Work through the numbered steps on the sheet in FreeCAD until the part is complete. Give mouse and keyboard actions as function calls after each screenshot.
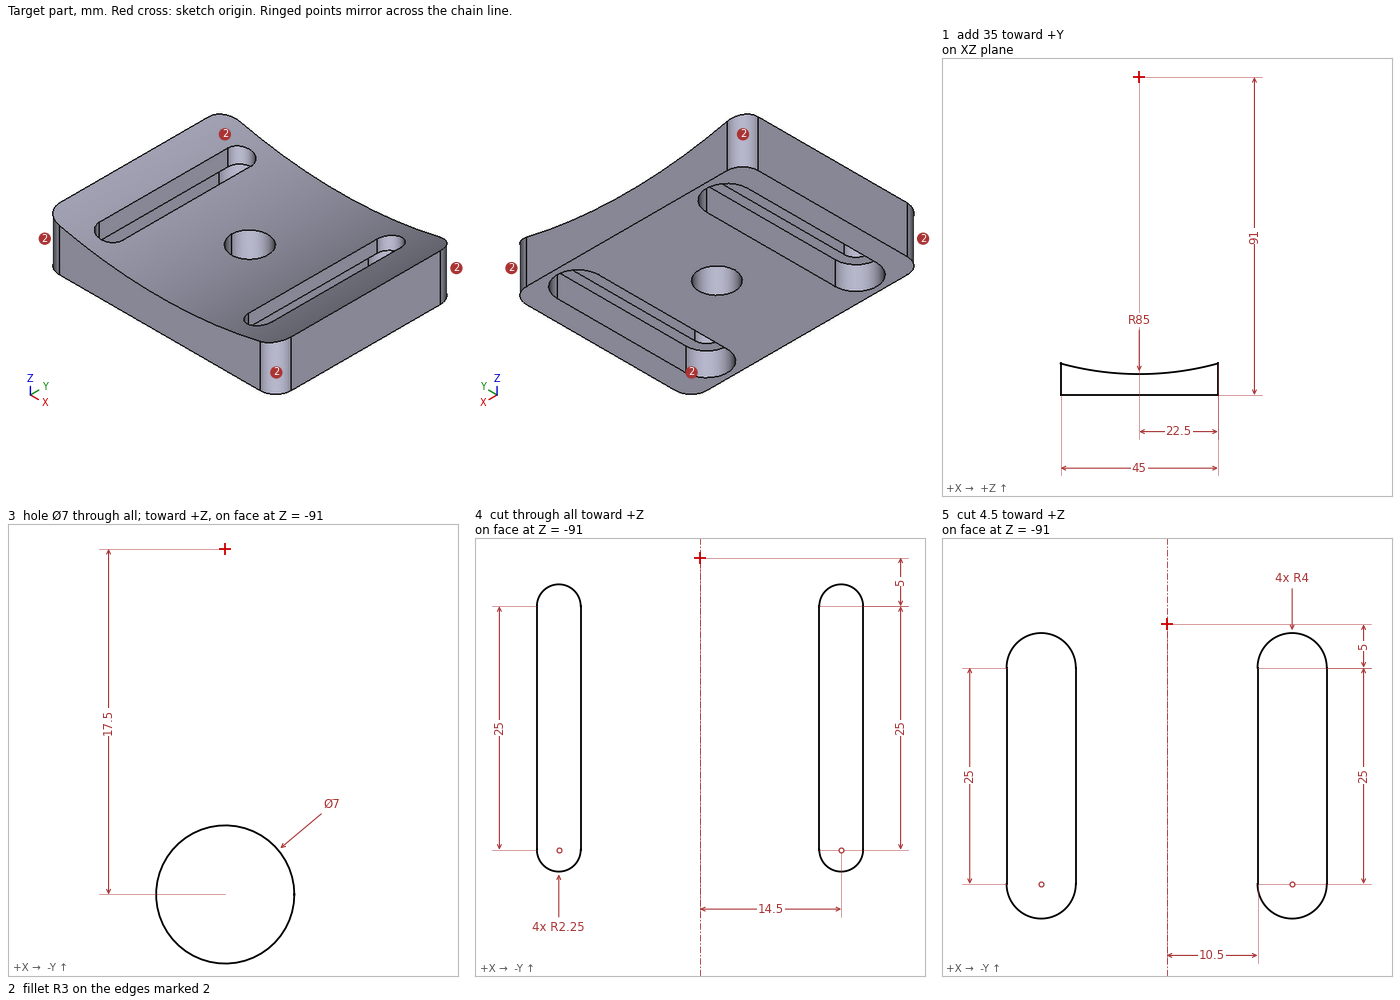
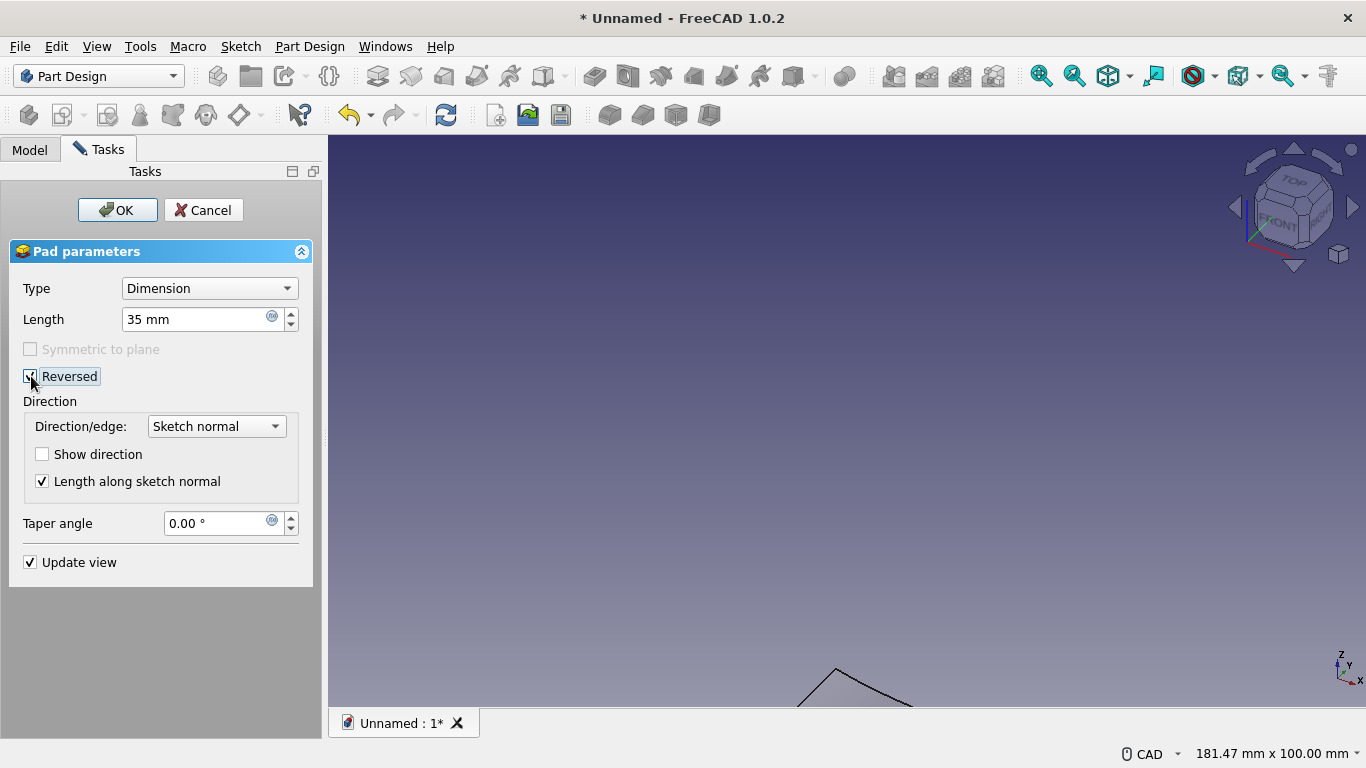
click(118, 210)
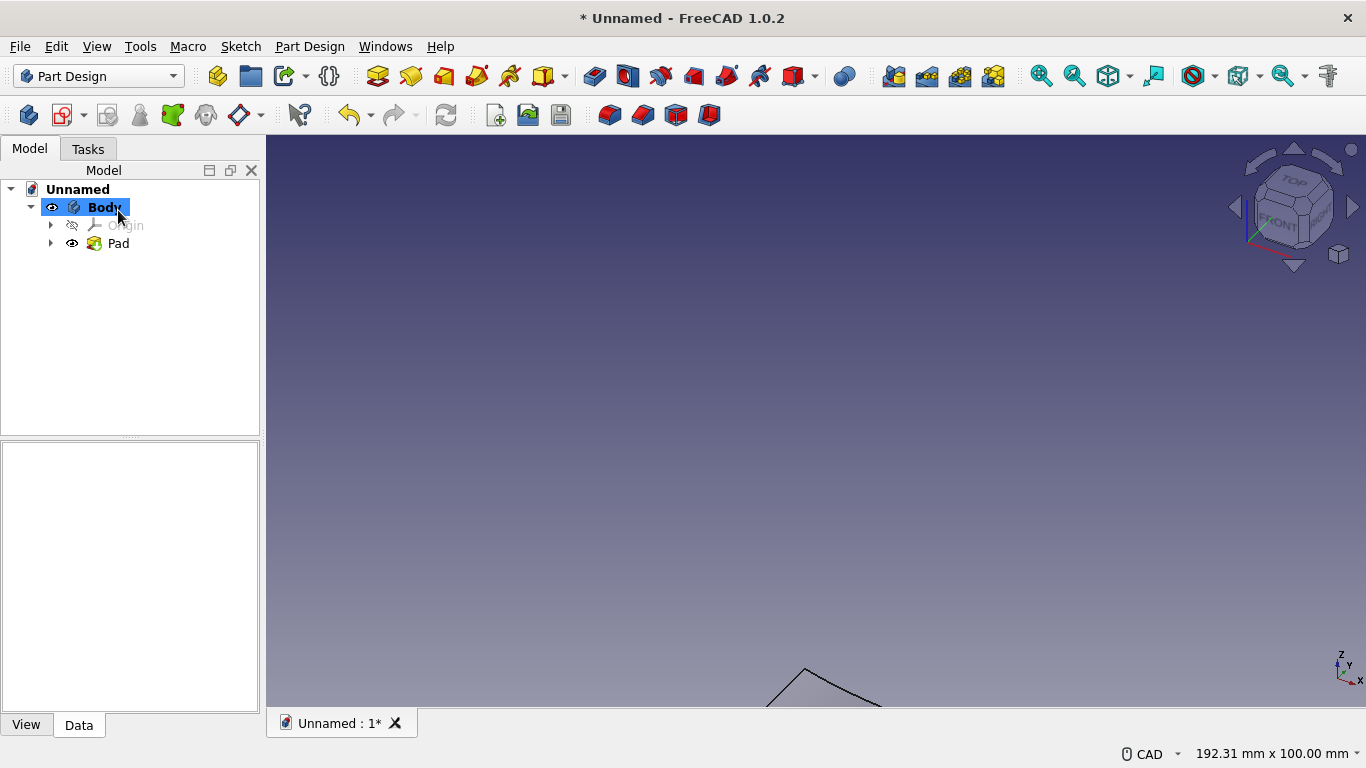
key(v)
key(f)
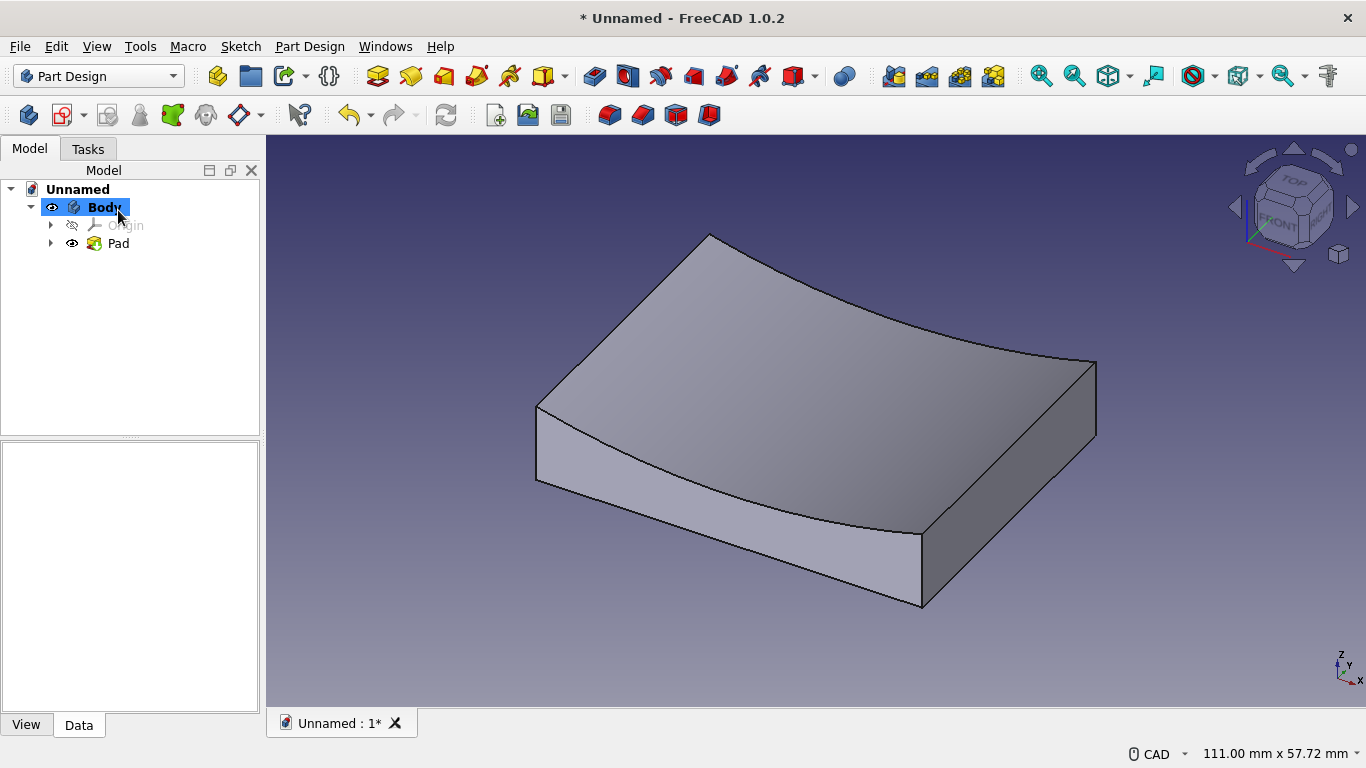
click(922, 570)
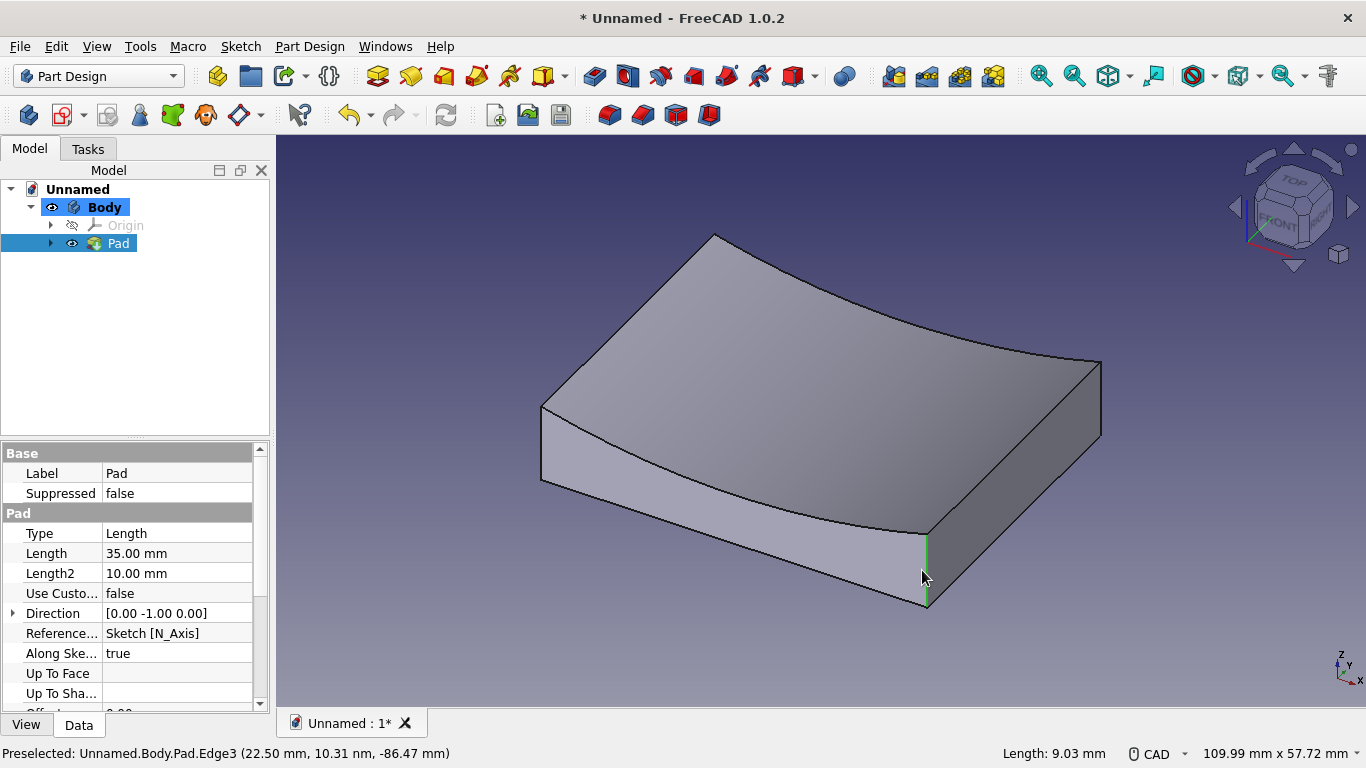
key(0)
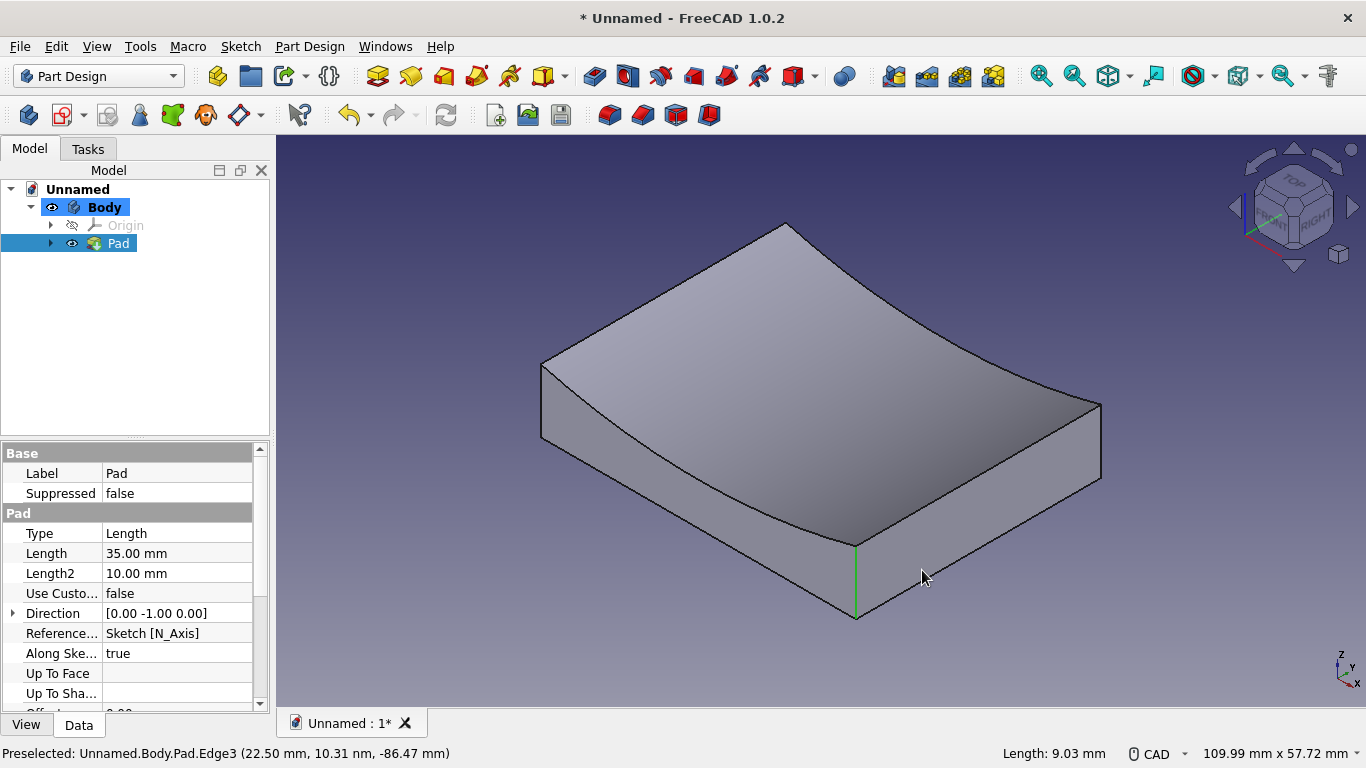
key(2)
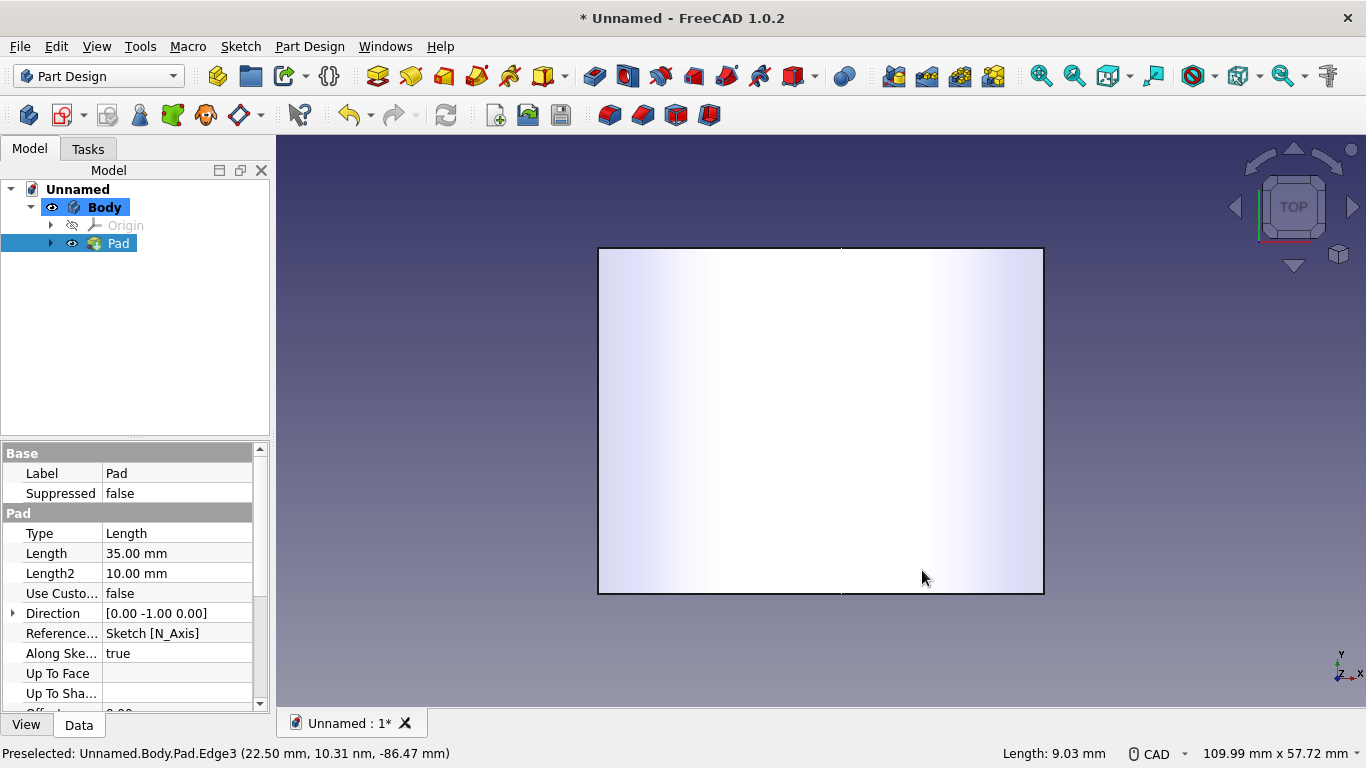
key(1)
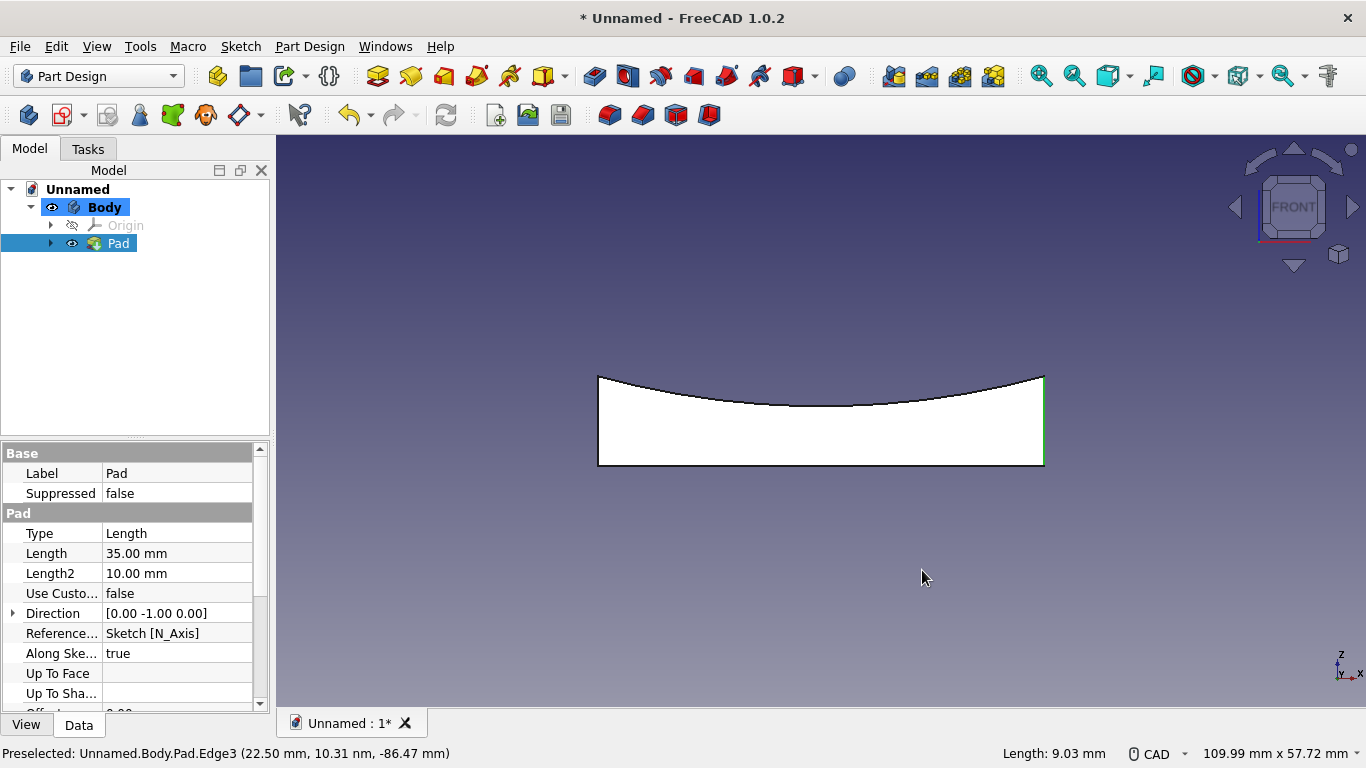
key(v)
key(f)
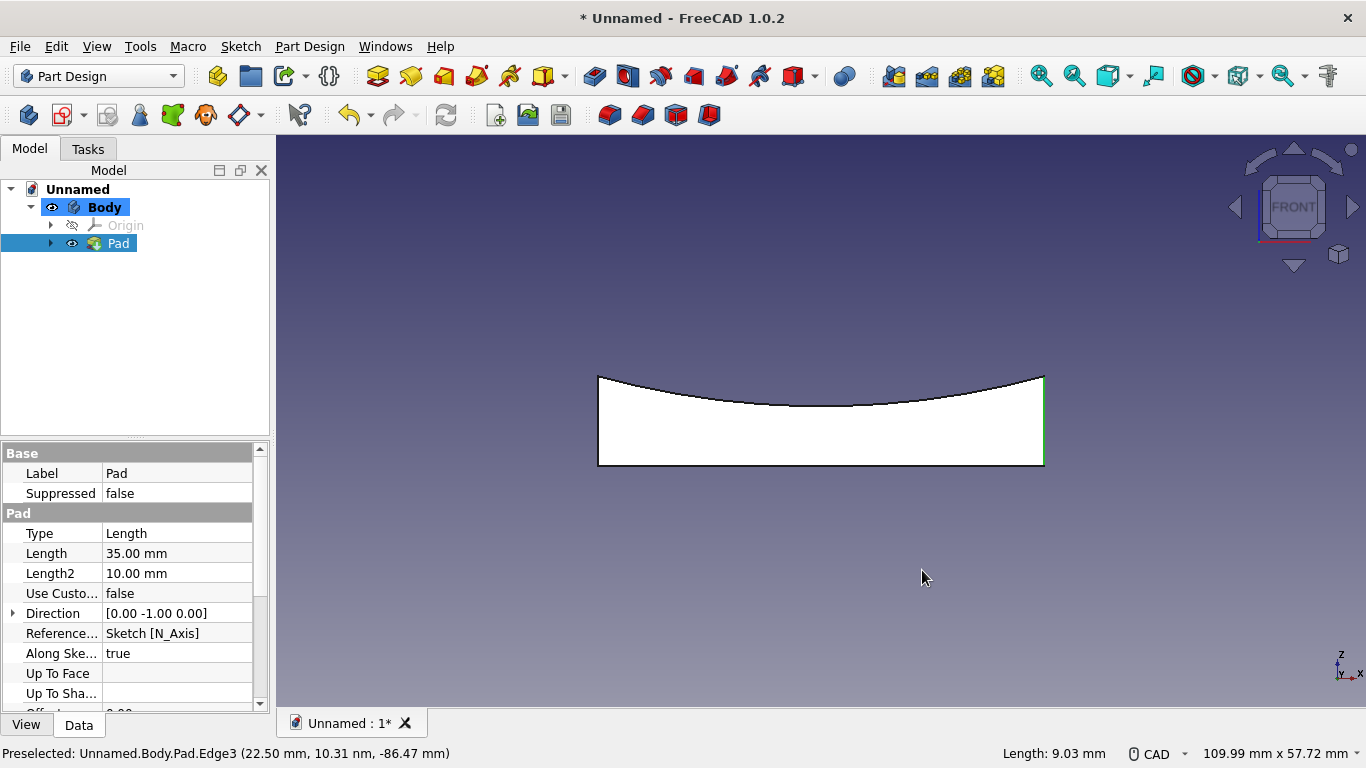
click(598, 429, ctrl)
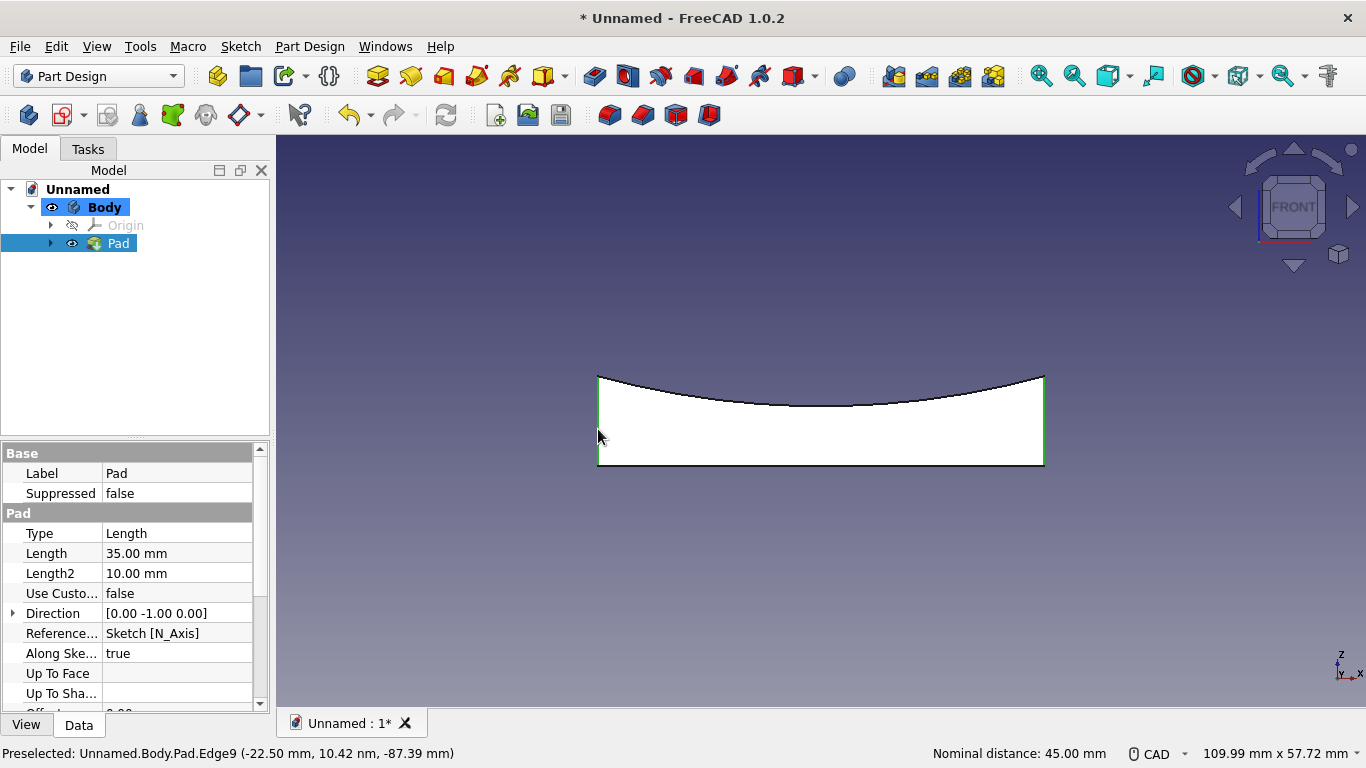
key(3)